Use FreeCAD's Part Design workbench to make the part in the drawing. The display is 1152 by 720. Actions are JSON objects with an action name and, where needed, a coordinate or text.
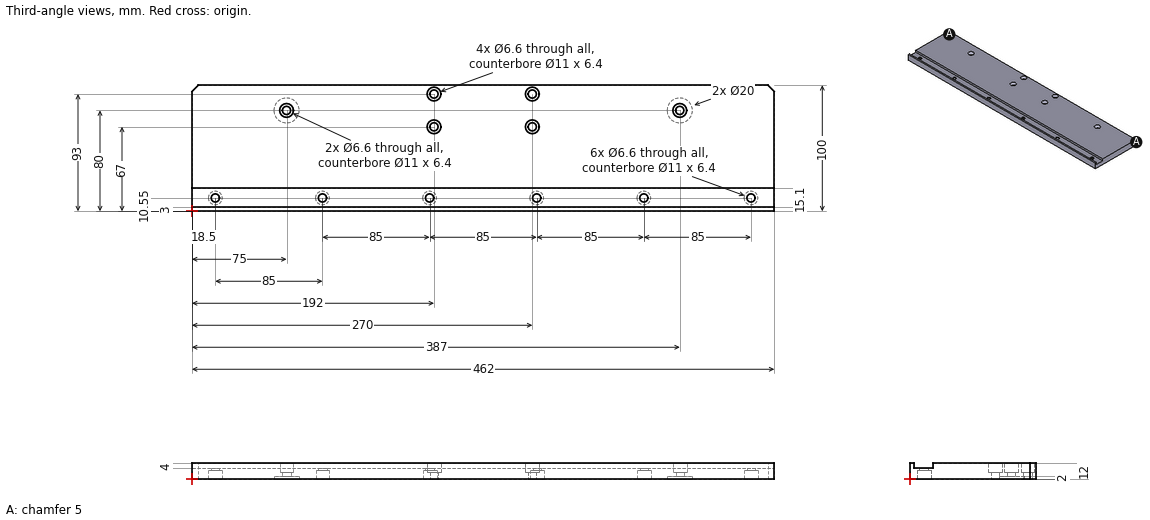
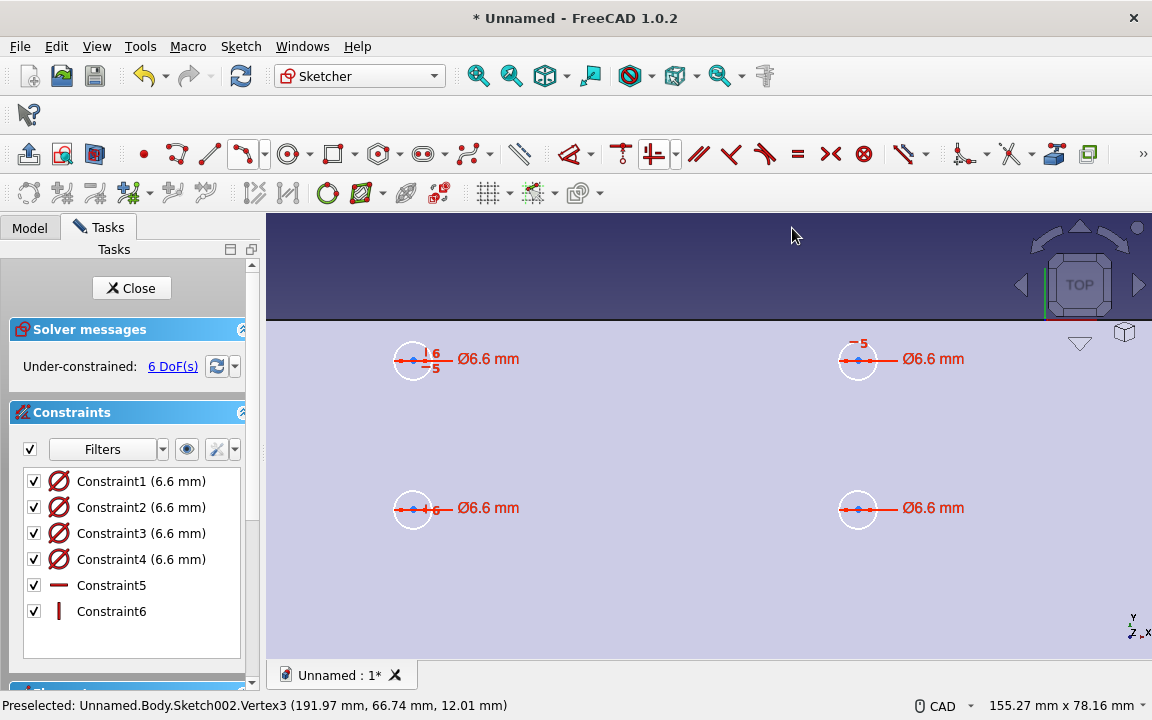
{"action": "left_click", "coordinate": [858, 361]}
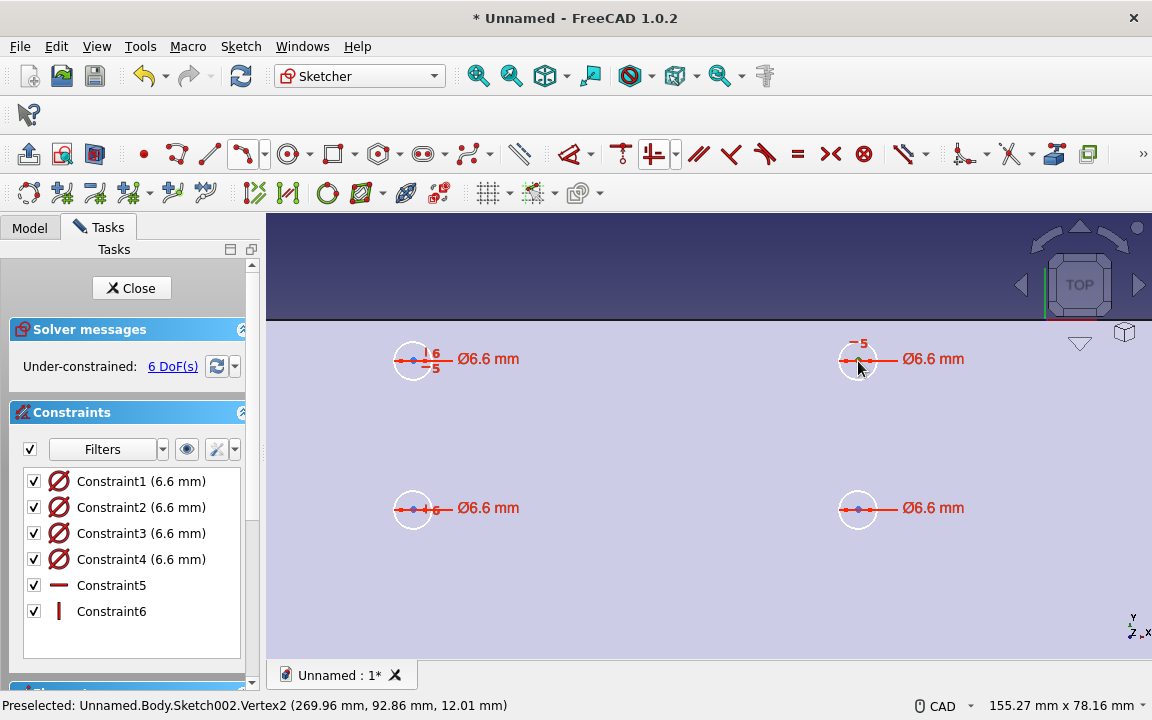
{"action": "left_click", "coordinate": [858, 510]}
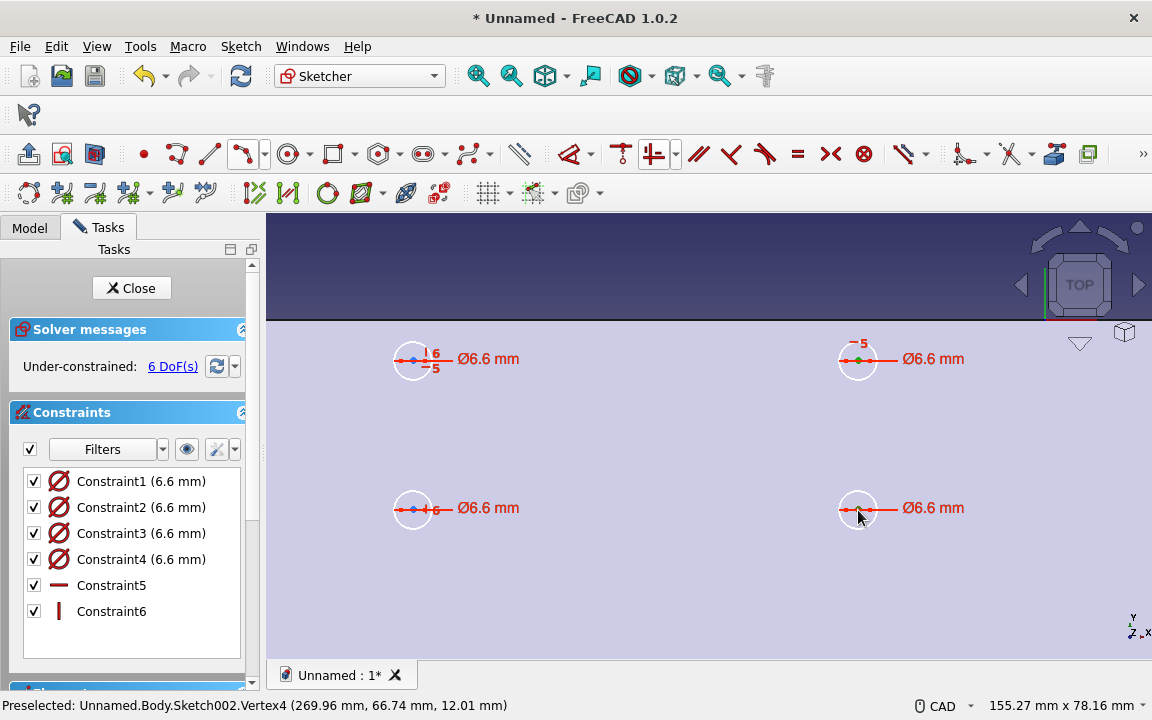
{"action": "left_click", "coordinate": [676, 154]}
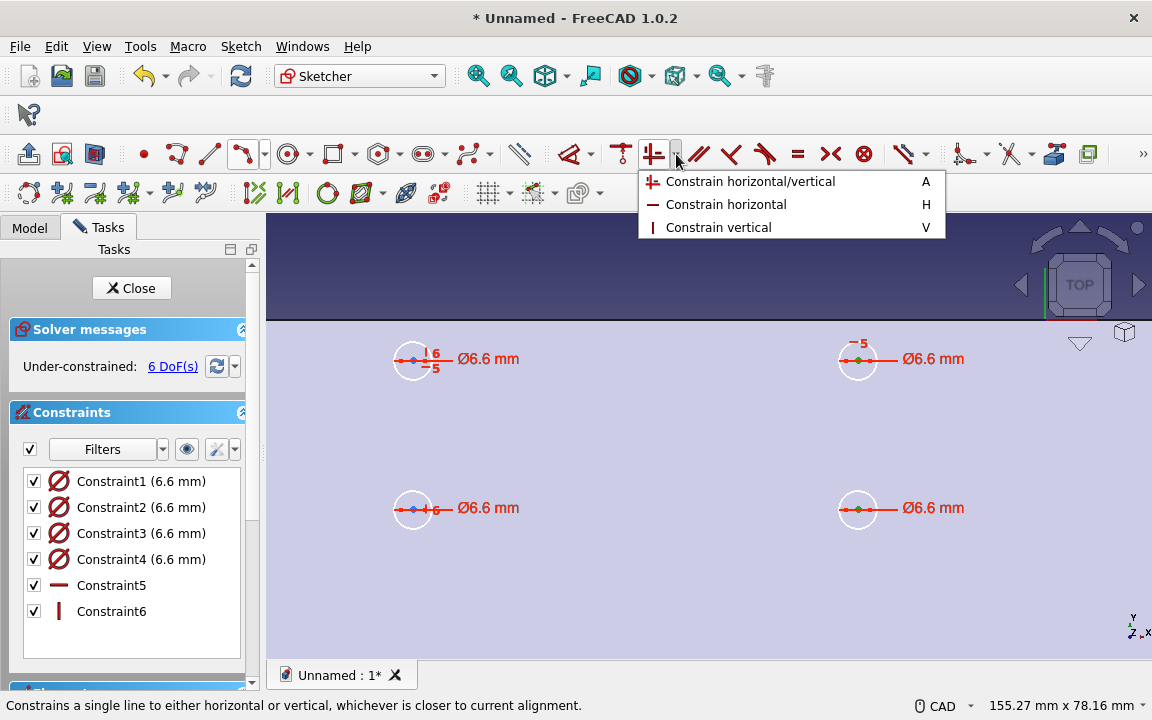
{"action": "left_click", "coordinate": [792, 228]}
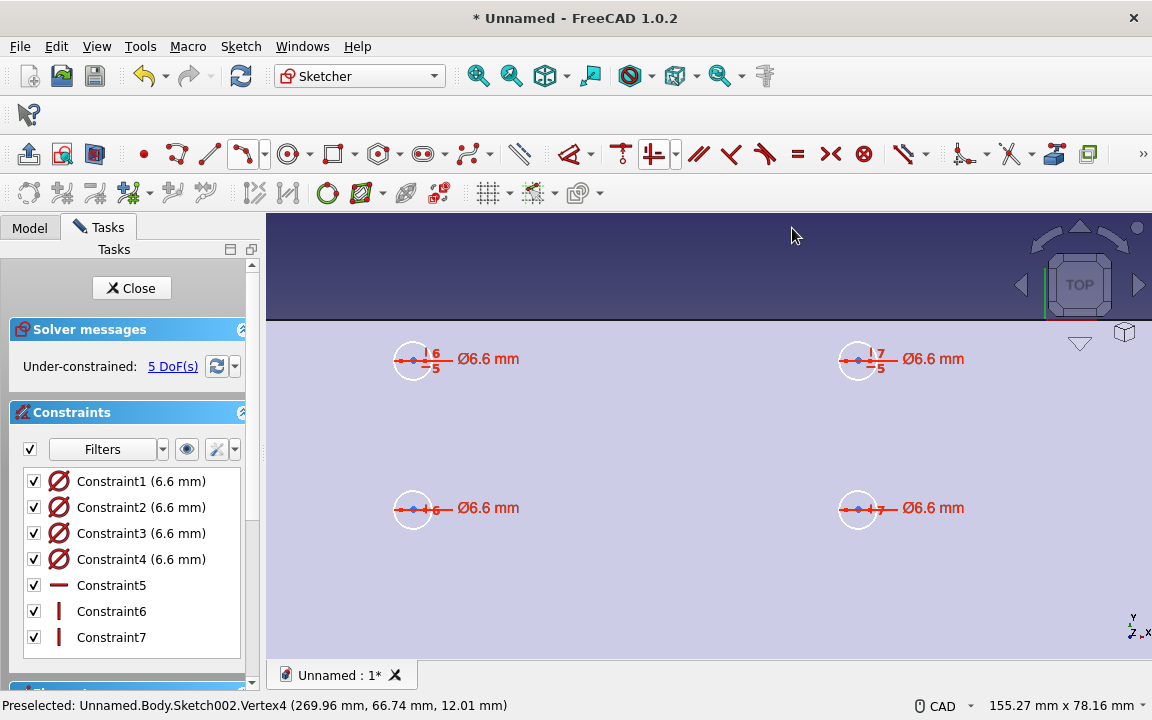
{"action": "left_click", "coordinate": [413, 510]}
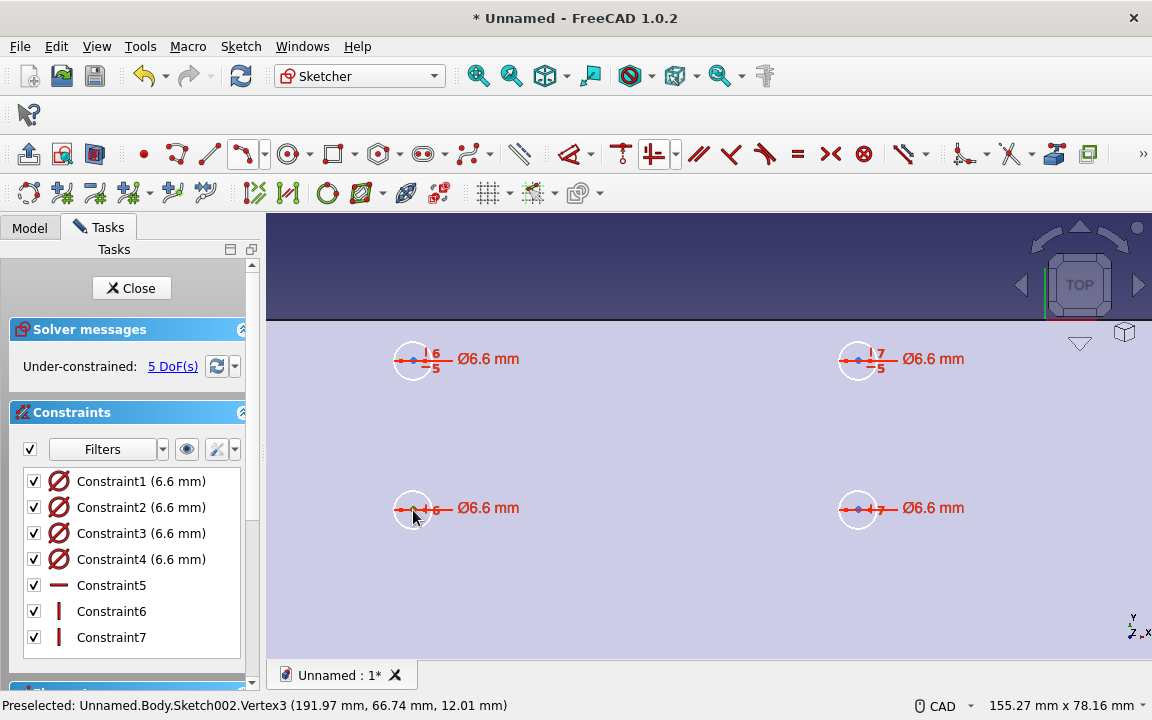
{"action": "left_click", "coordinate": [858, 510]}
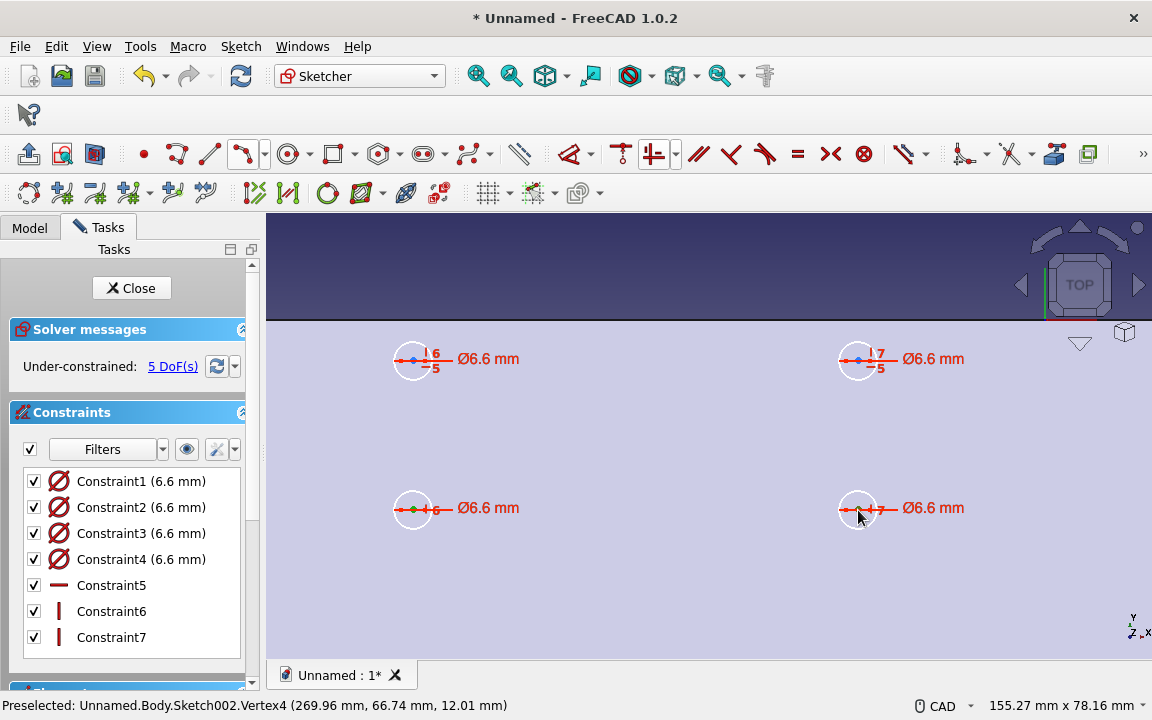
{"action": "key", "text": "h"}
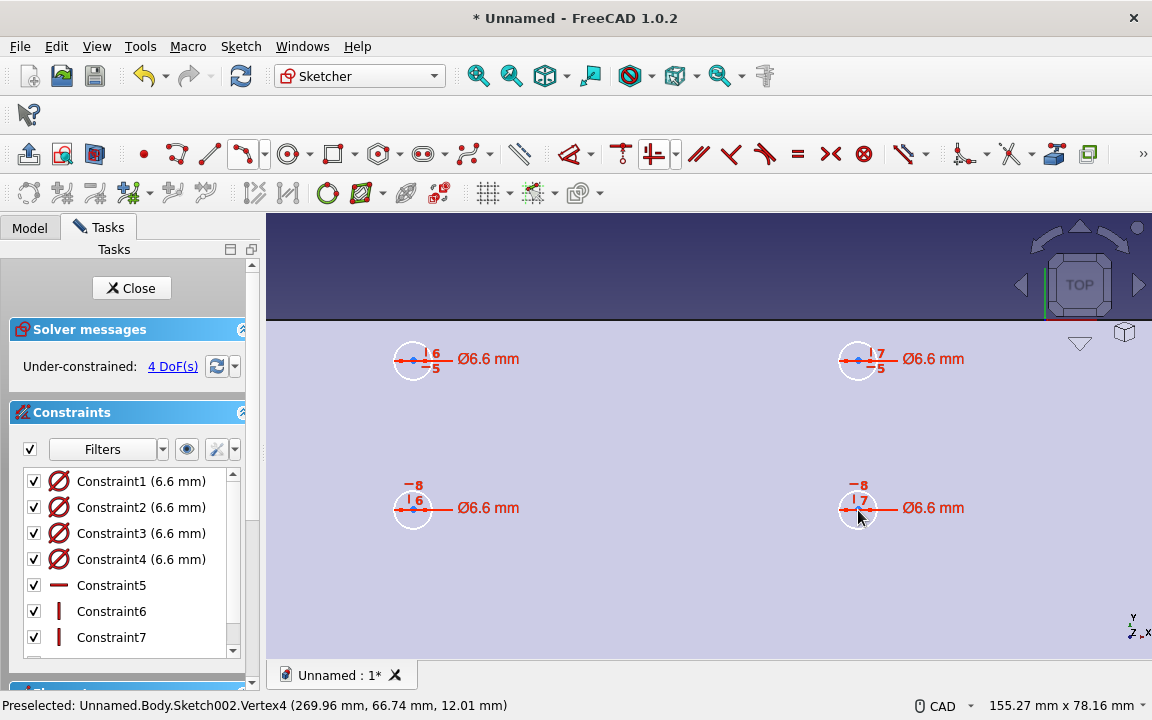
{"action": "left_click", "coordinate": [568, 154]}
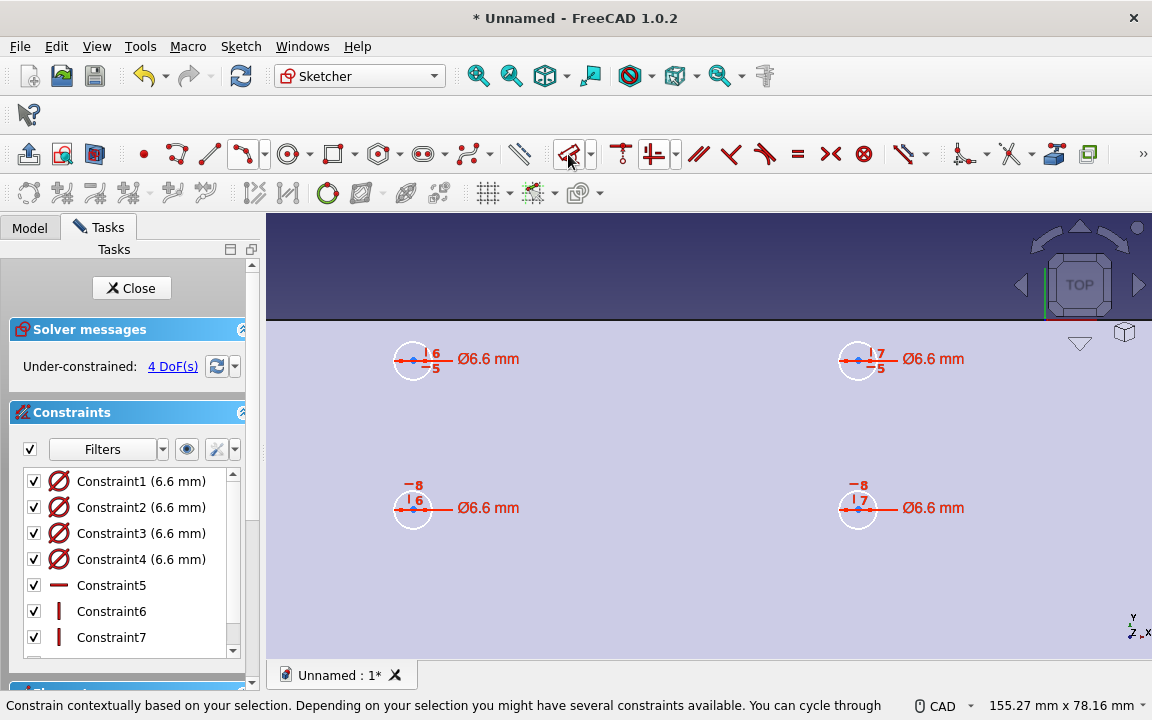
{"action": "left_click", "coordinate": [413, 361]}
{"action": "left_click", "coordinate": [447, 496]}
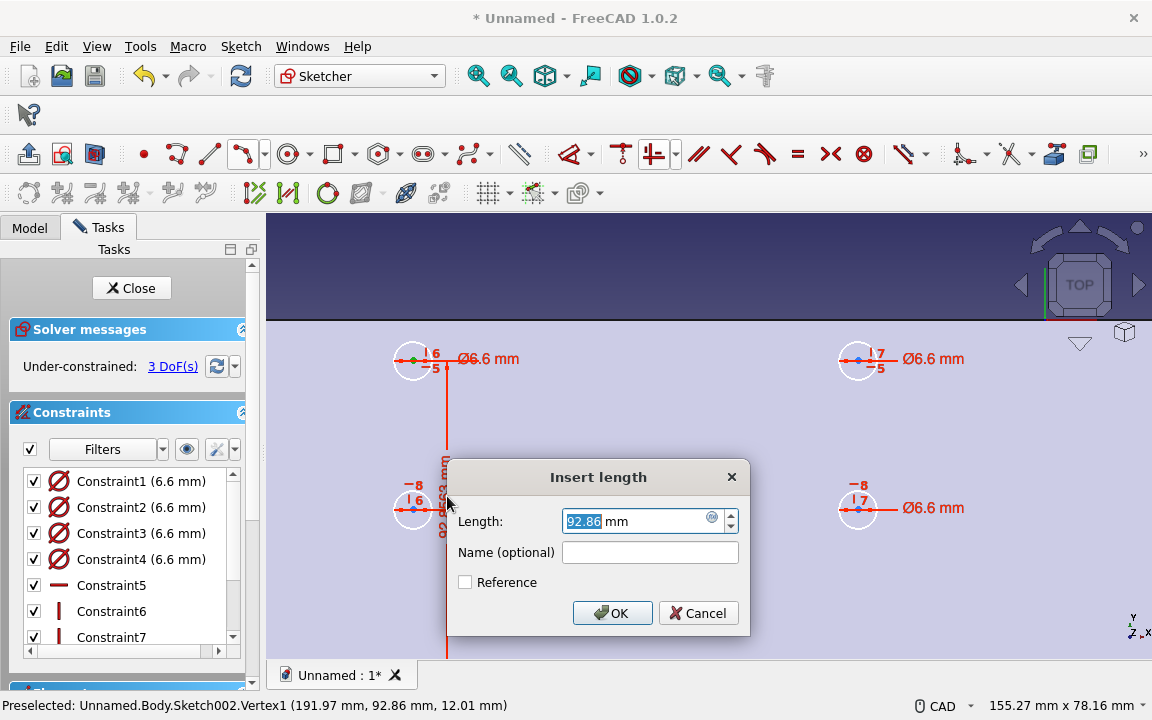
{"action": "type", "text": "93"}
{"action": "key", "text": "Return"}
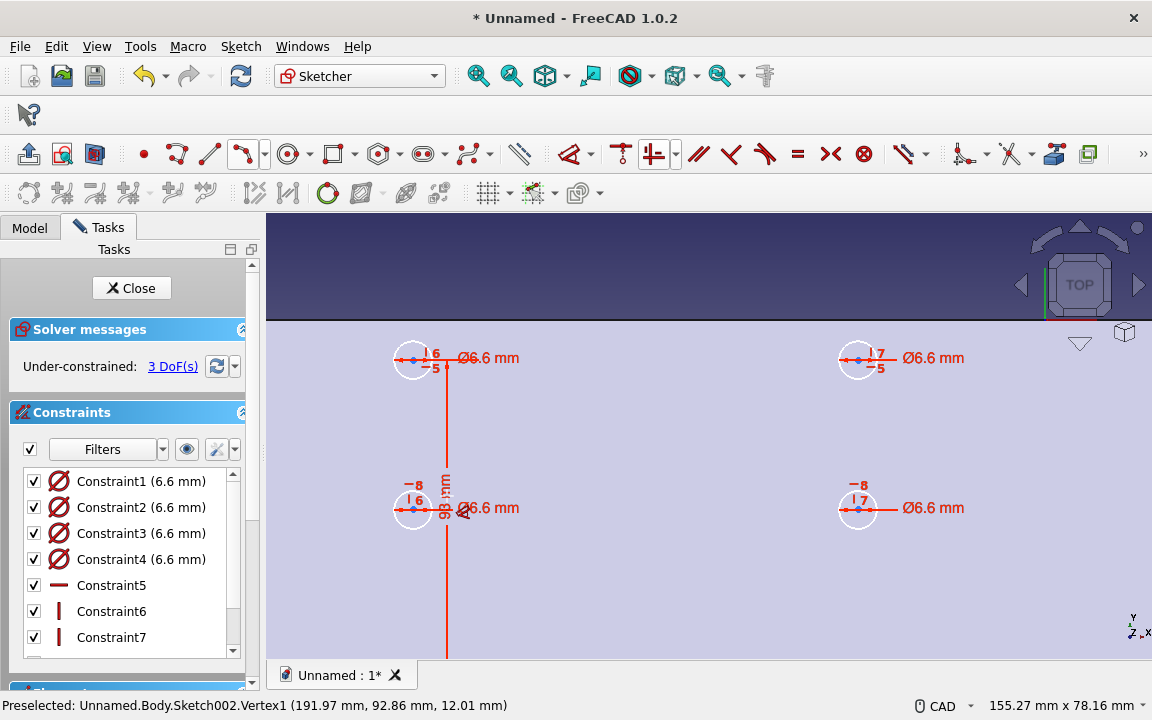
{"action": "left_click", "coordinate": [413, 510]}
{"action": "left_click", "coordinate": [447, 571]}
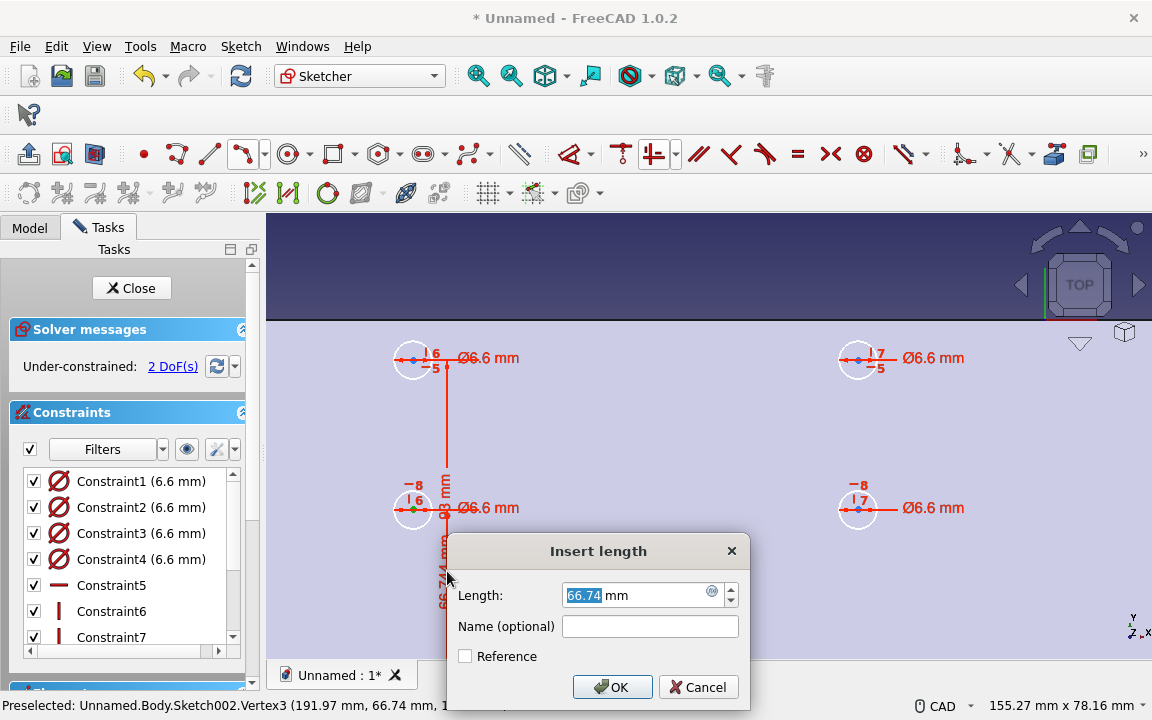
{"action": "type", "text": "67"}
{"action": "key", "text": "Return"}